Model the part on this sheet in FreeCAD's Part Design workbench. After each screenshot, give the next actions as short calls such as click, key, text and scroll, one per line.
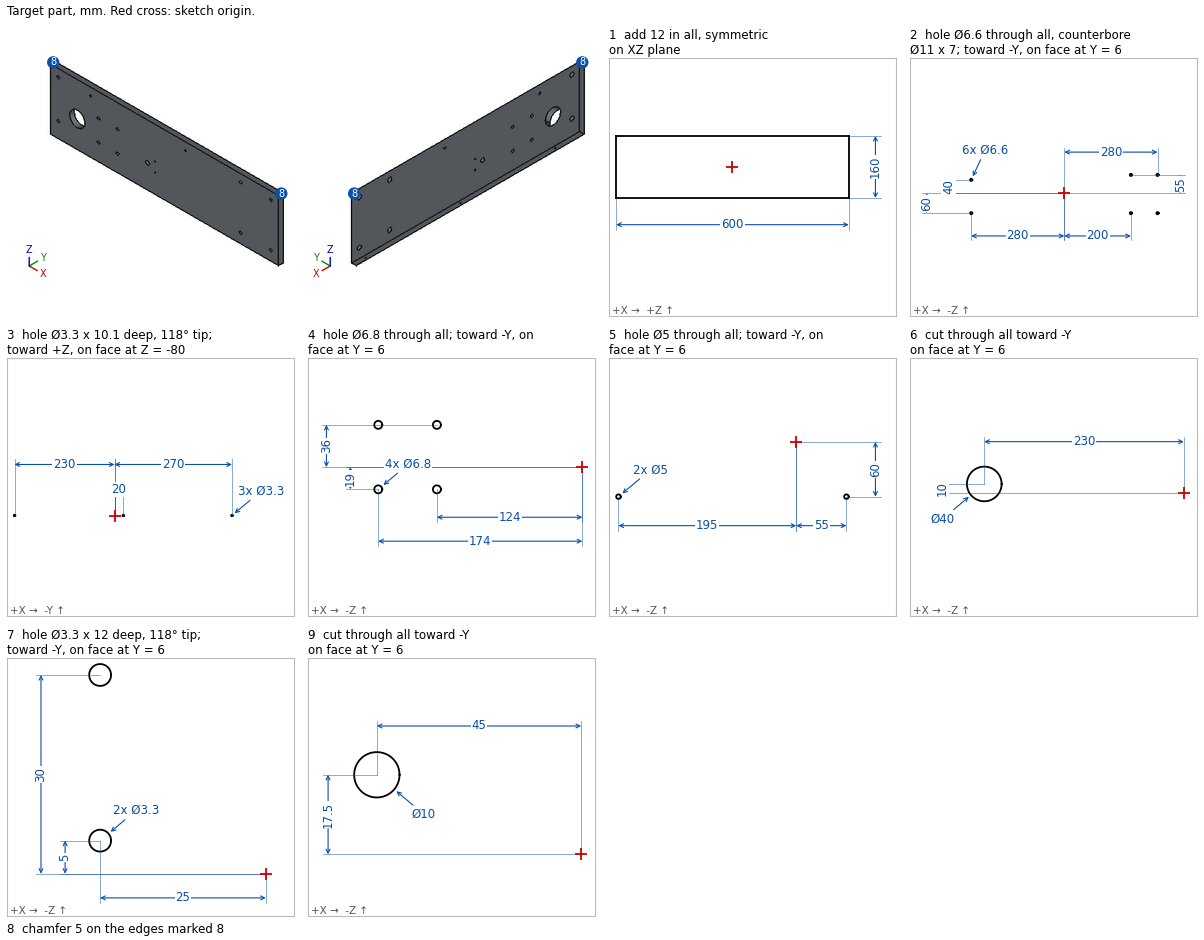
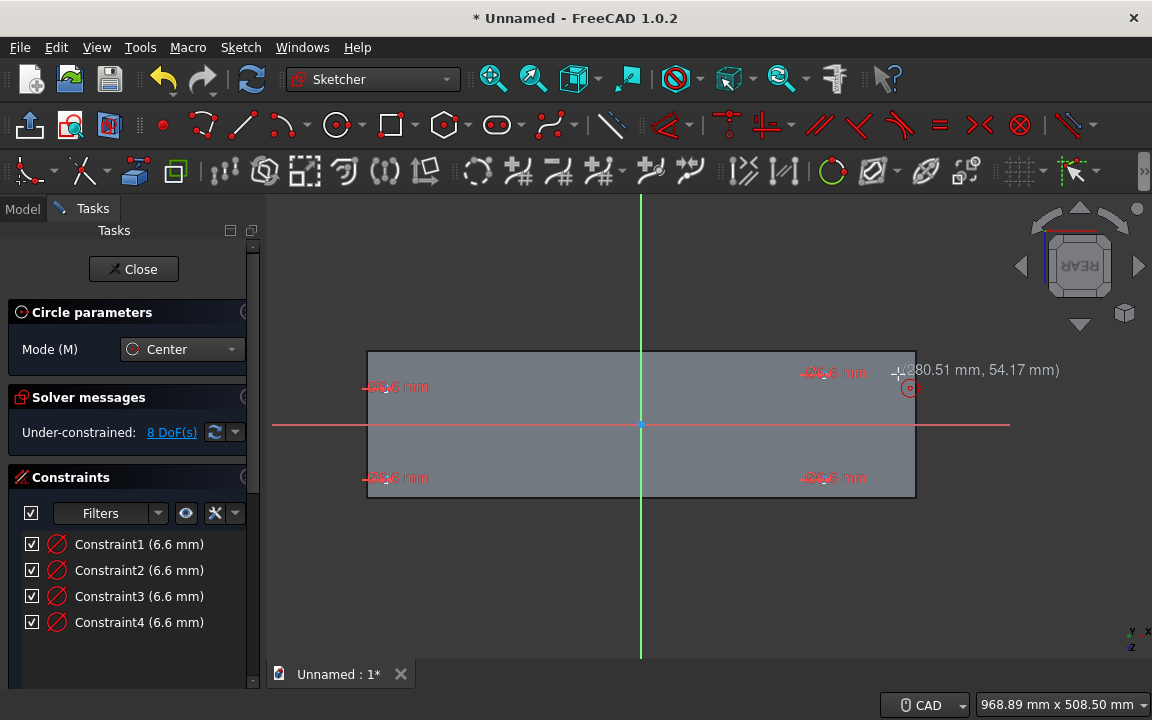
click(898, 374)
move(900, 372)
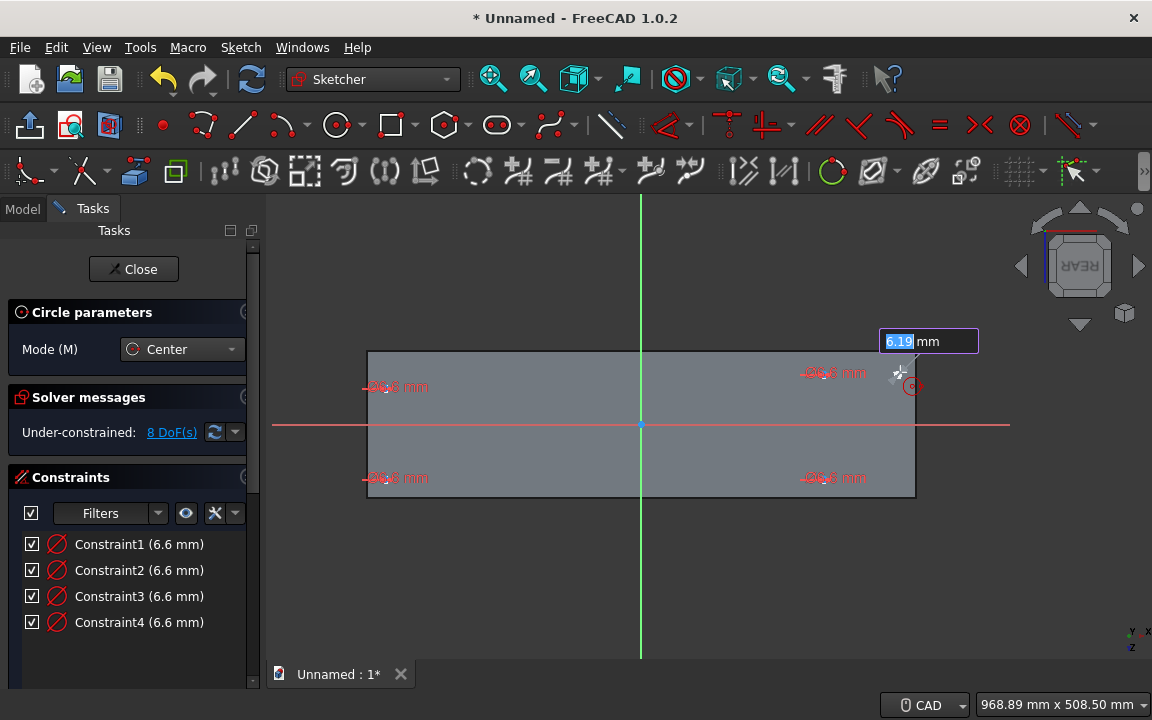
text(6.6)
key(Return)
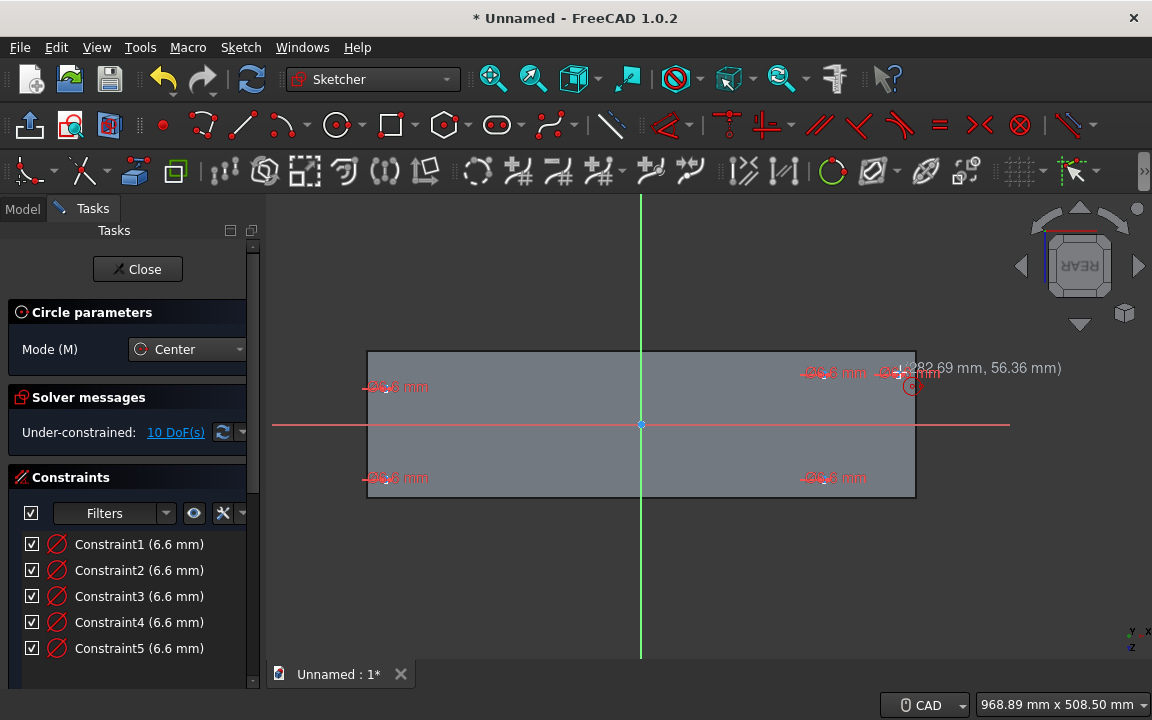
scroll(898, 479, up, 11)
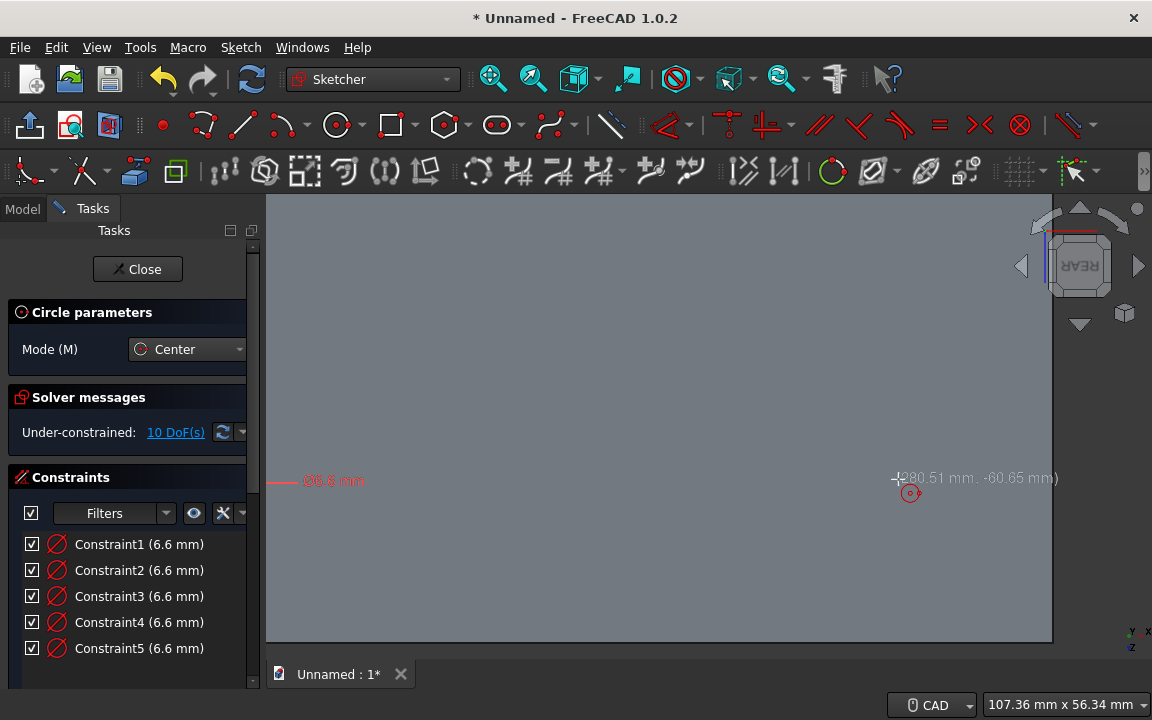
scroll(898, 479, down, 11)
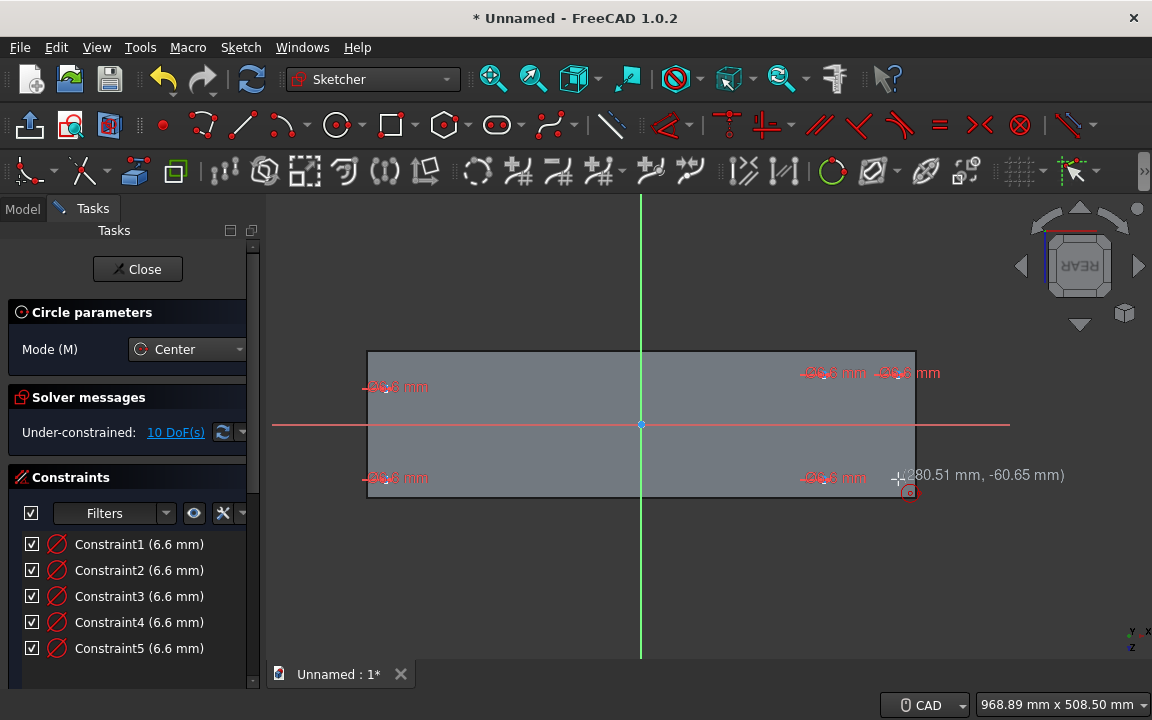
click(898, 479)
move(900, 477)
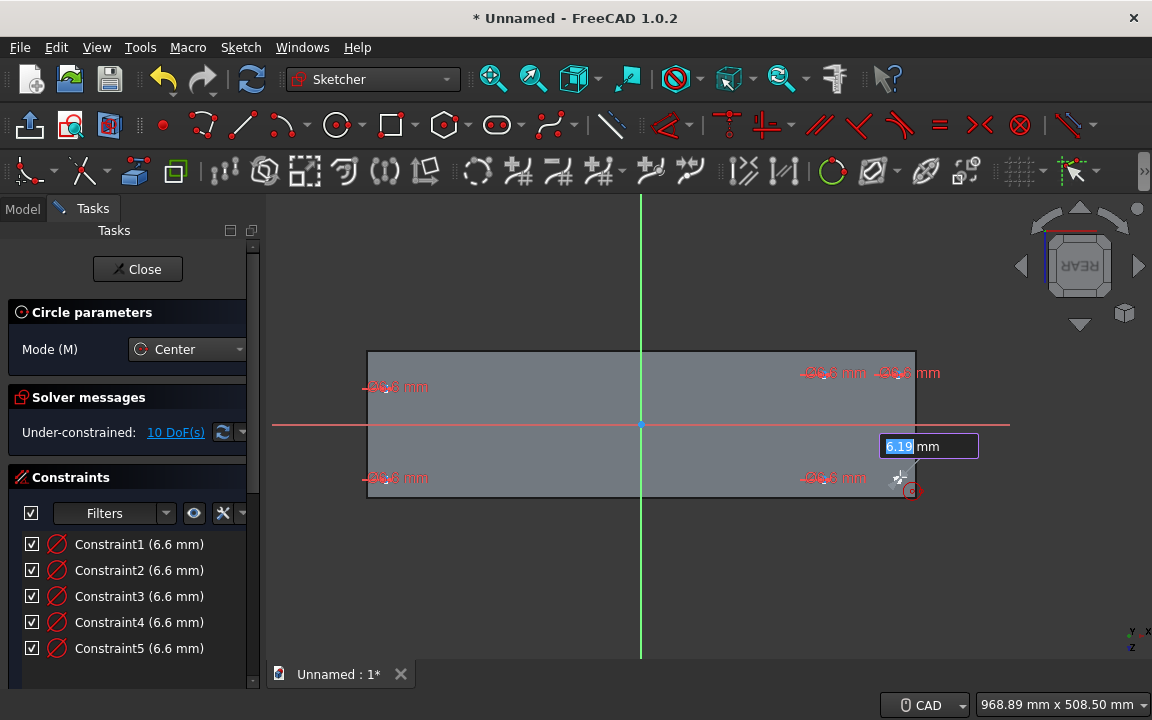
text(6.6)
key(Return)
key(Escape)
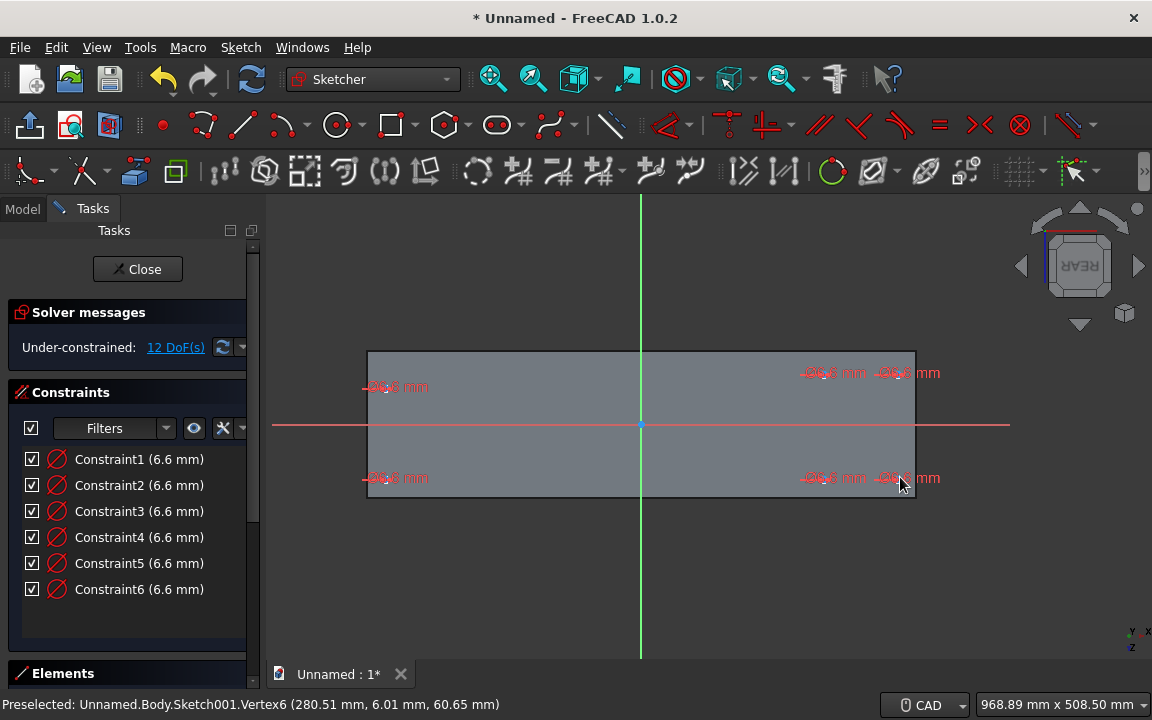
click(386, 480)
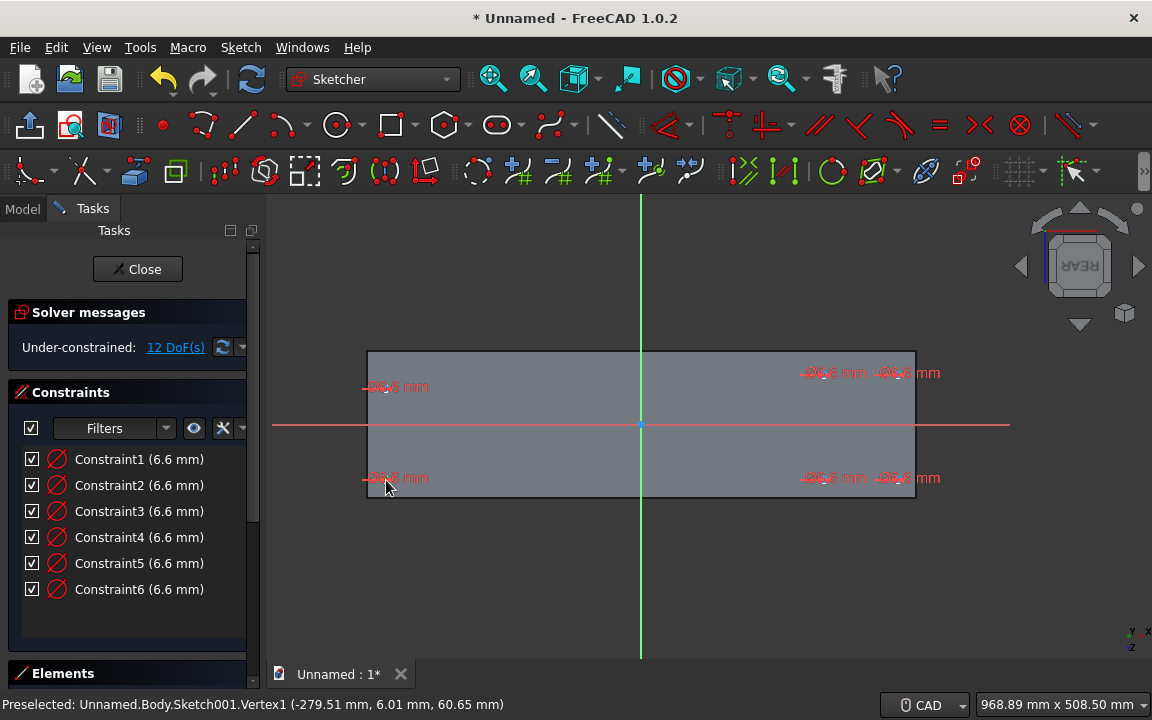
click(386, 389)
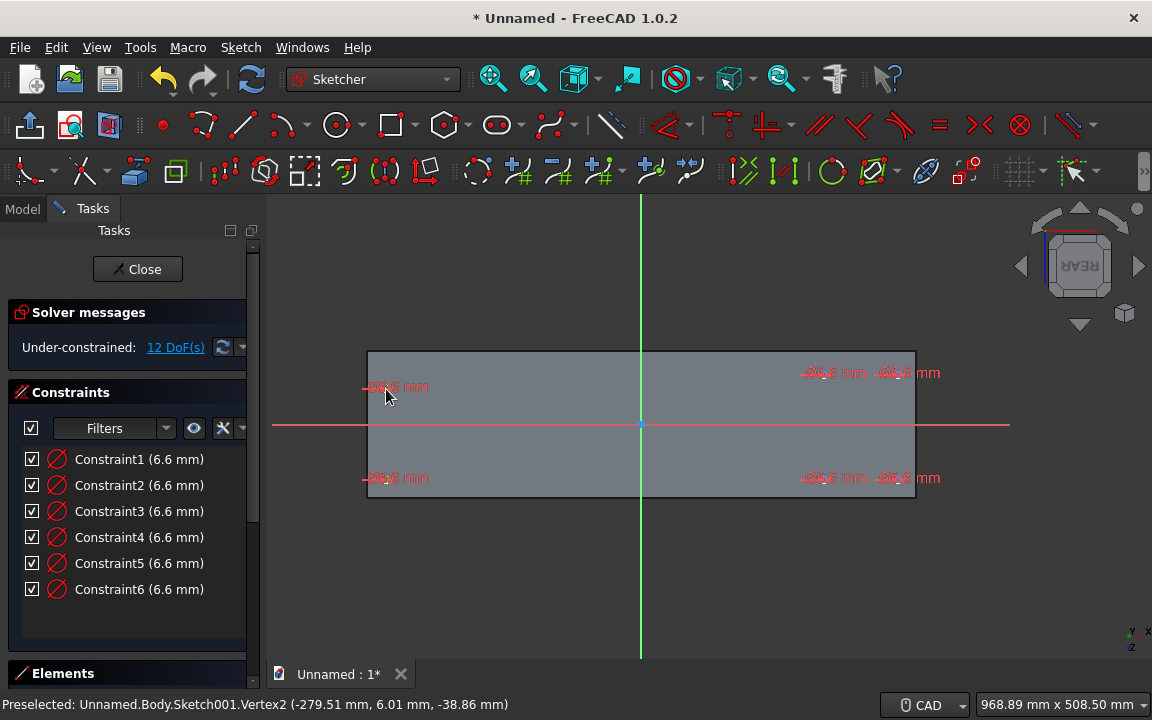
click(794, 126)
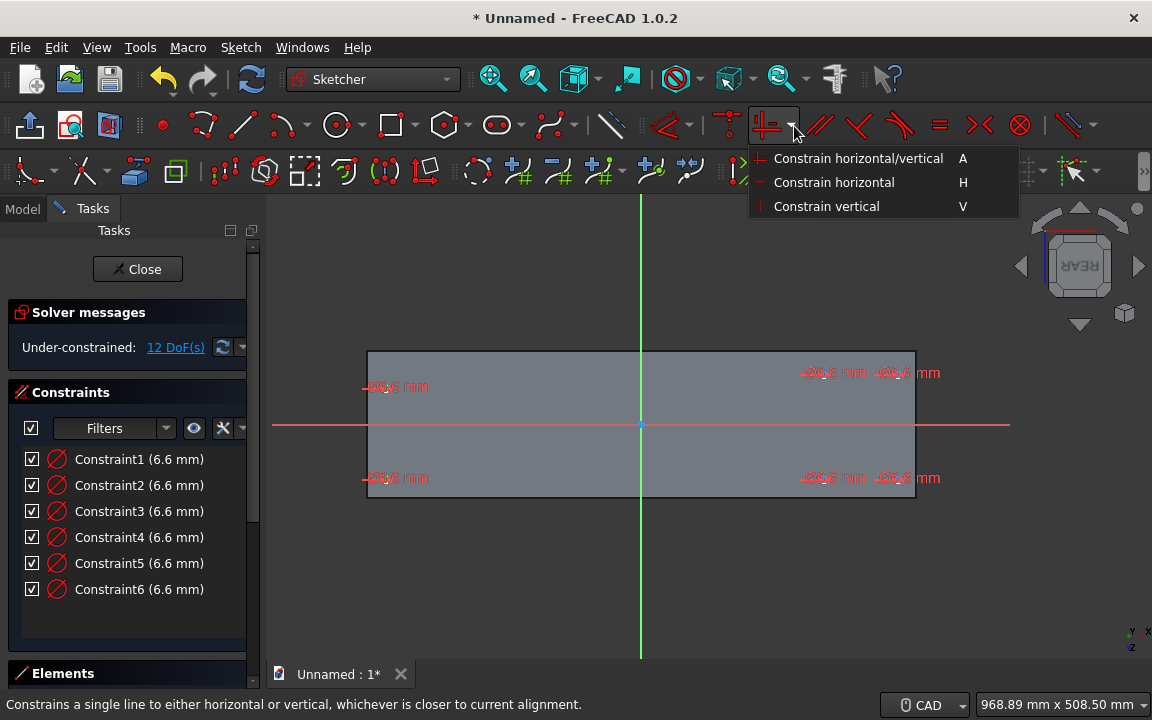
click(884, 206)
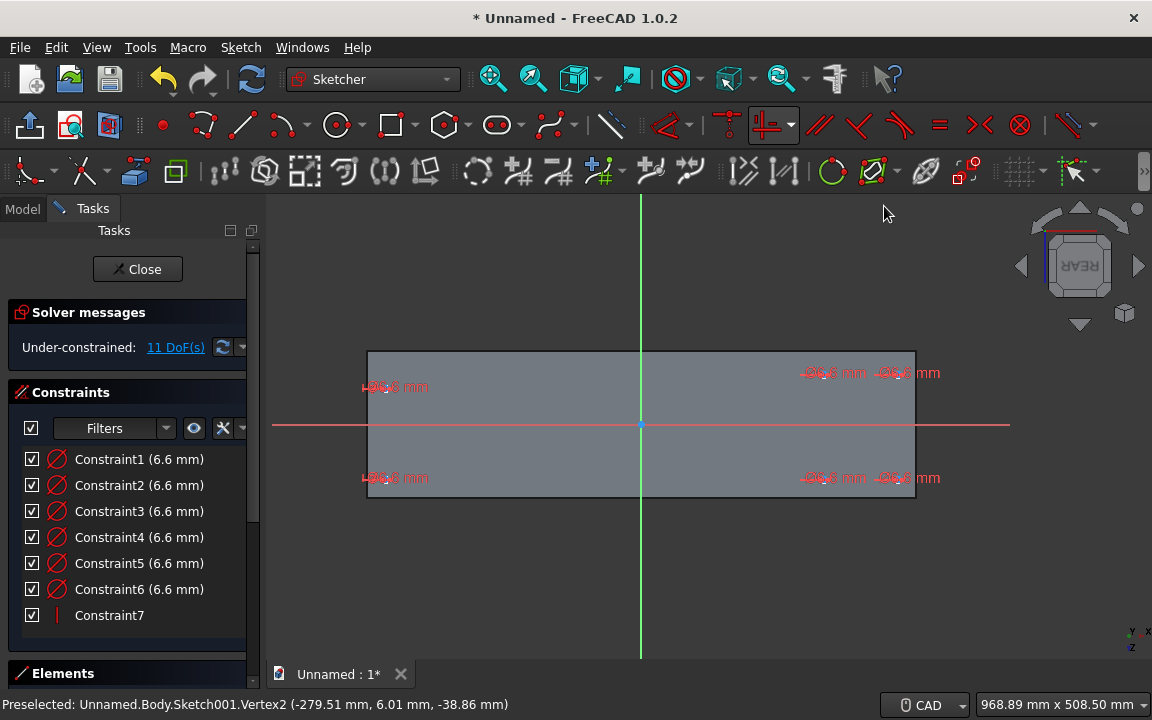
click(386, 480)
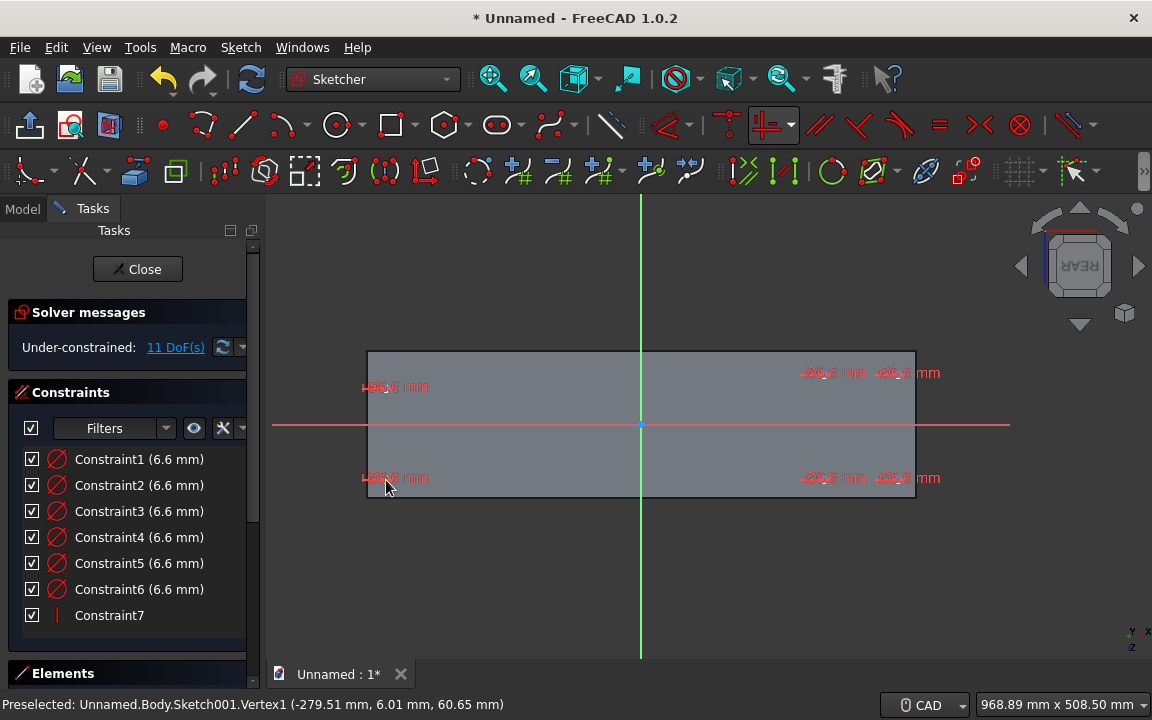
click(824, 480)